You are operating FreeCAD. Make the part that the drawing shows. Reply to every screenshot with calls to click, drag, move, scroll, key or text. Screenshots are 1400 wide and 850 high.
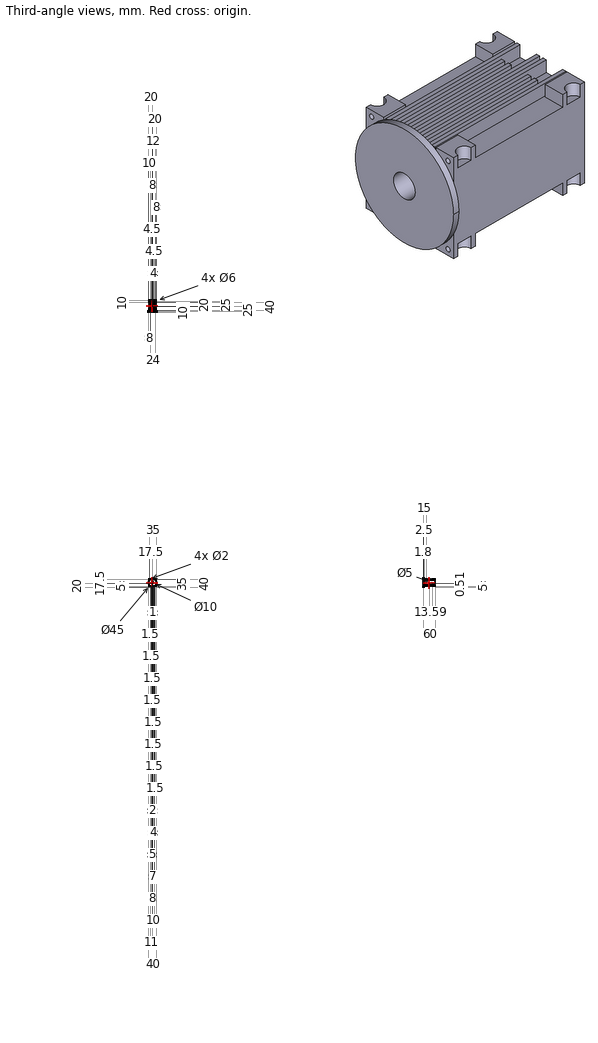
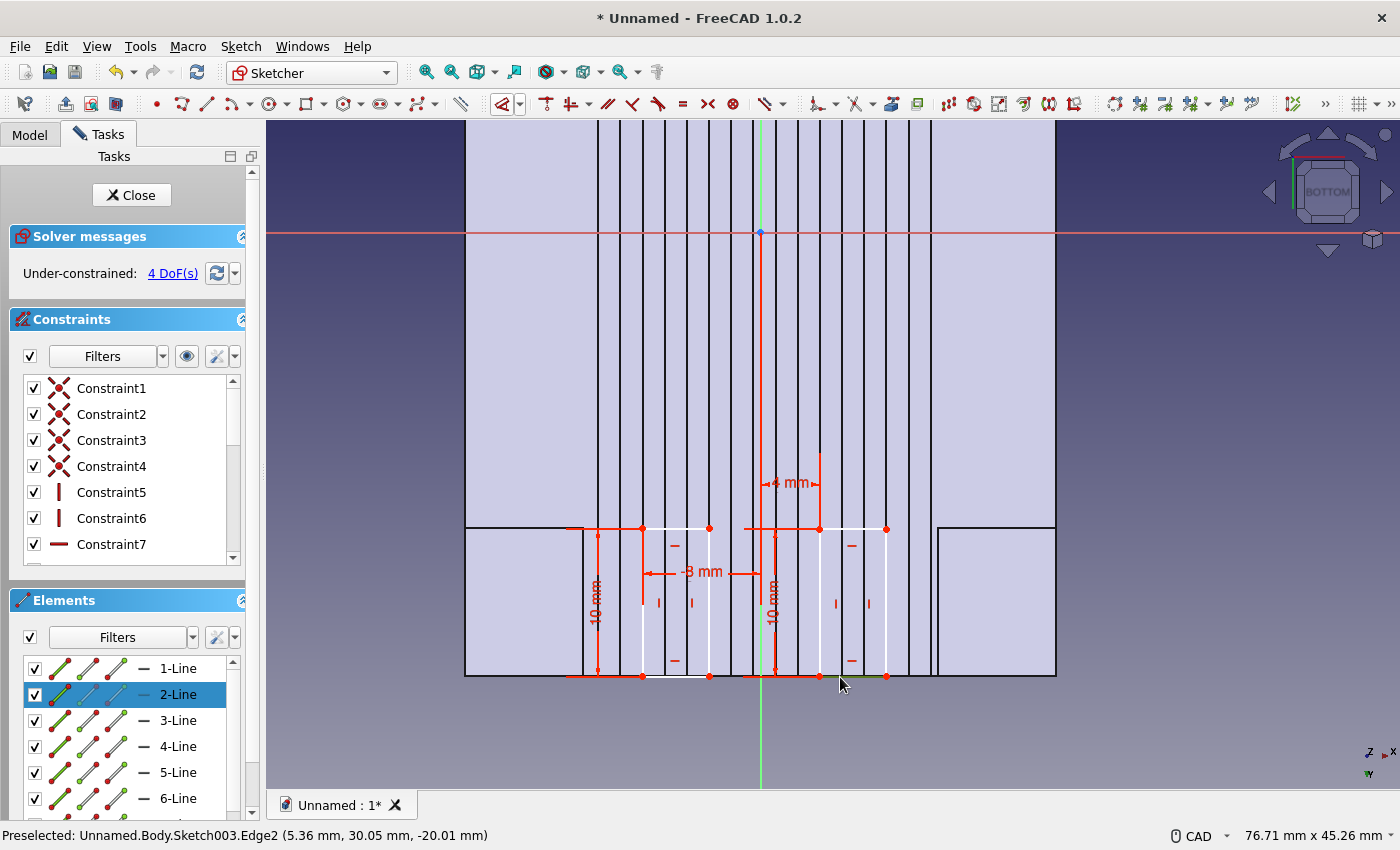
key(l)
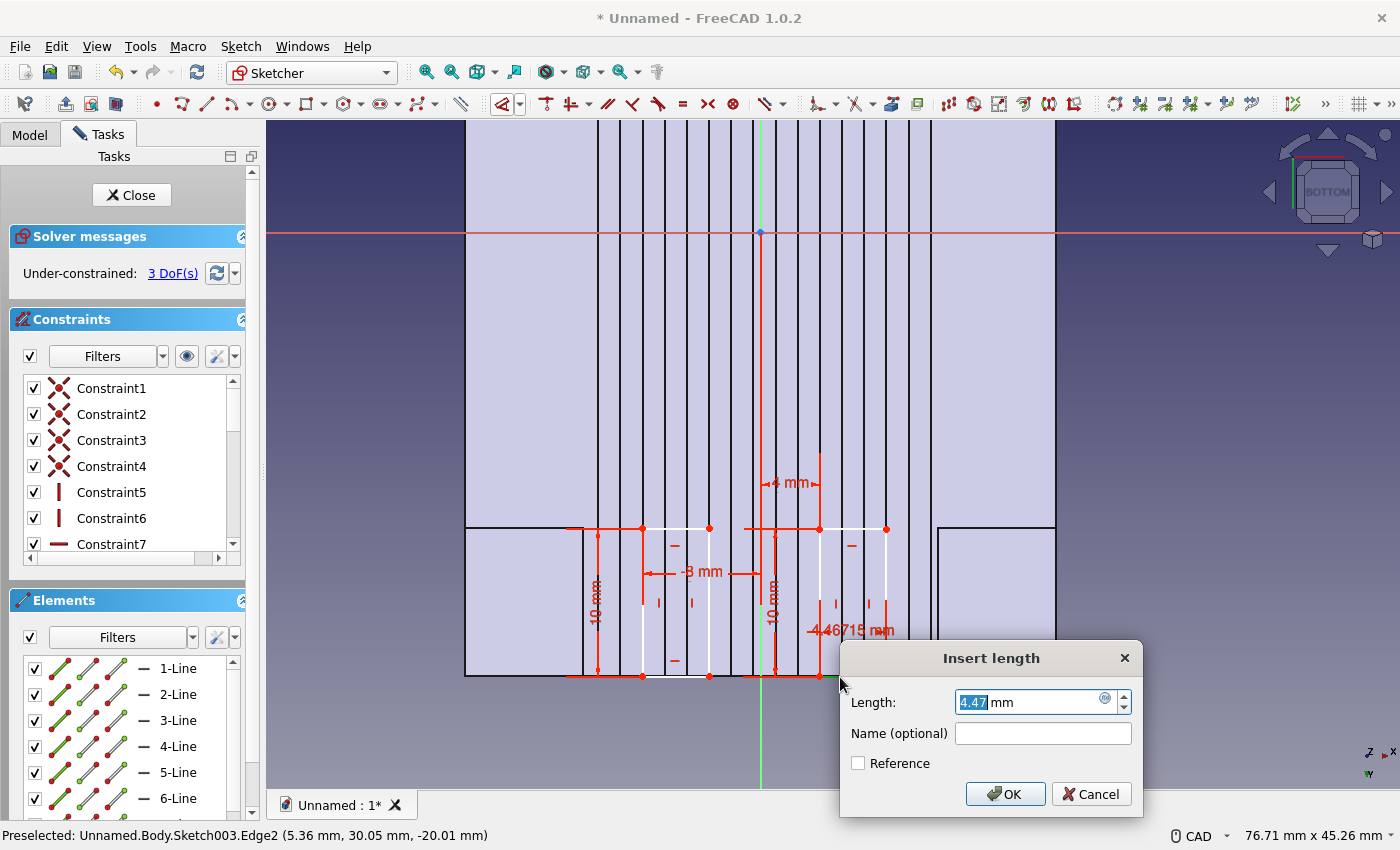
text(4.5)
key(Return)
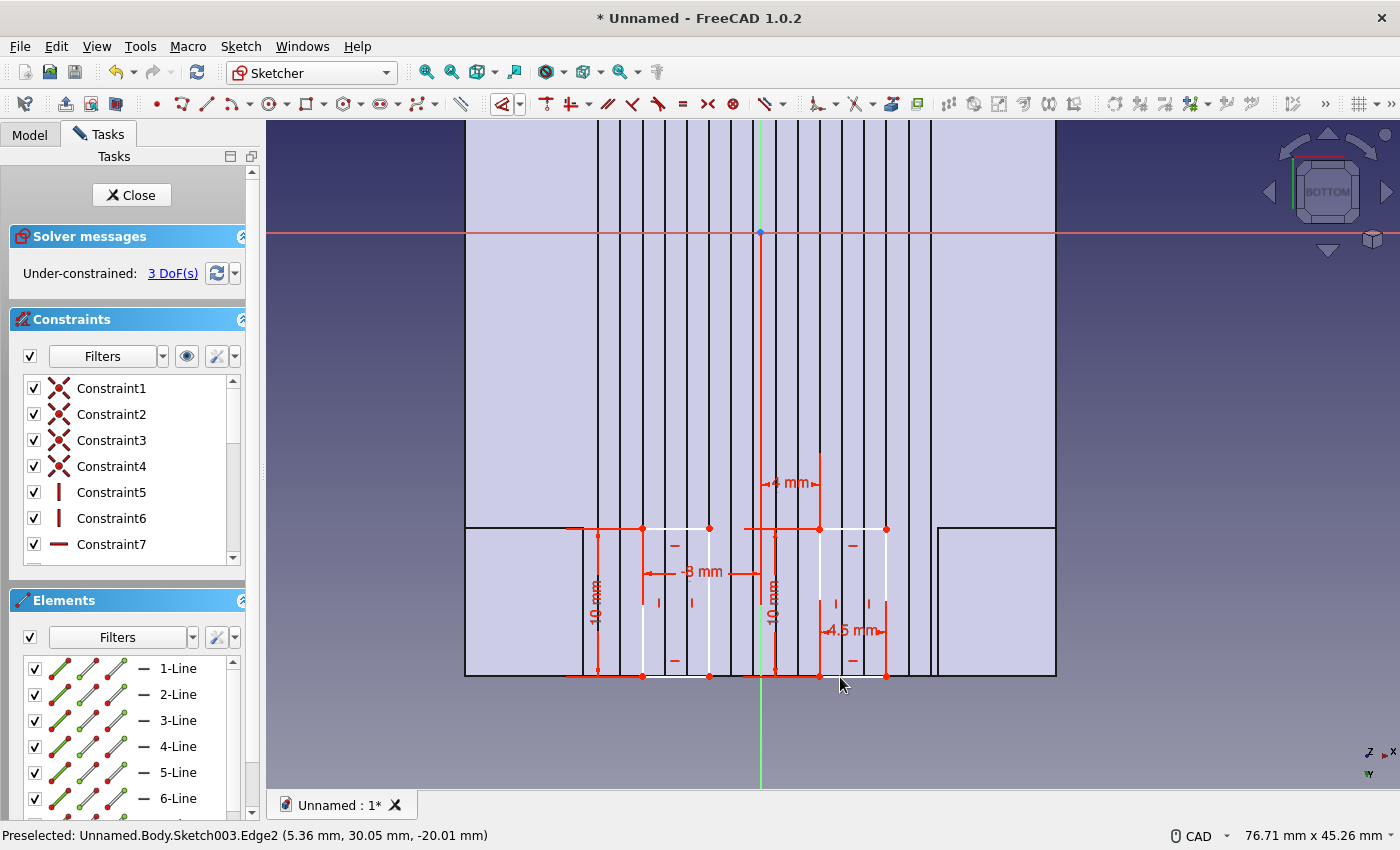
click(663, 677)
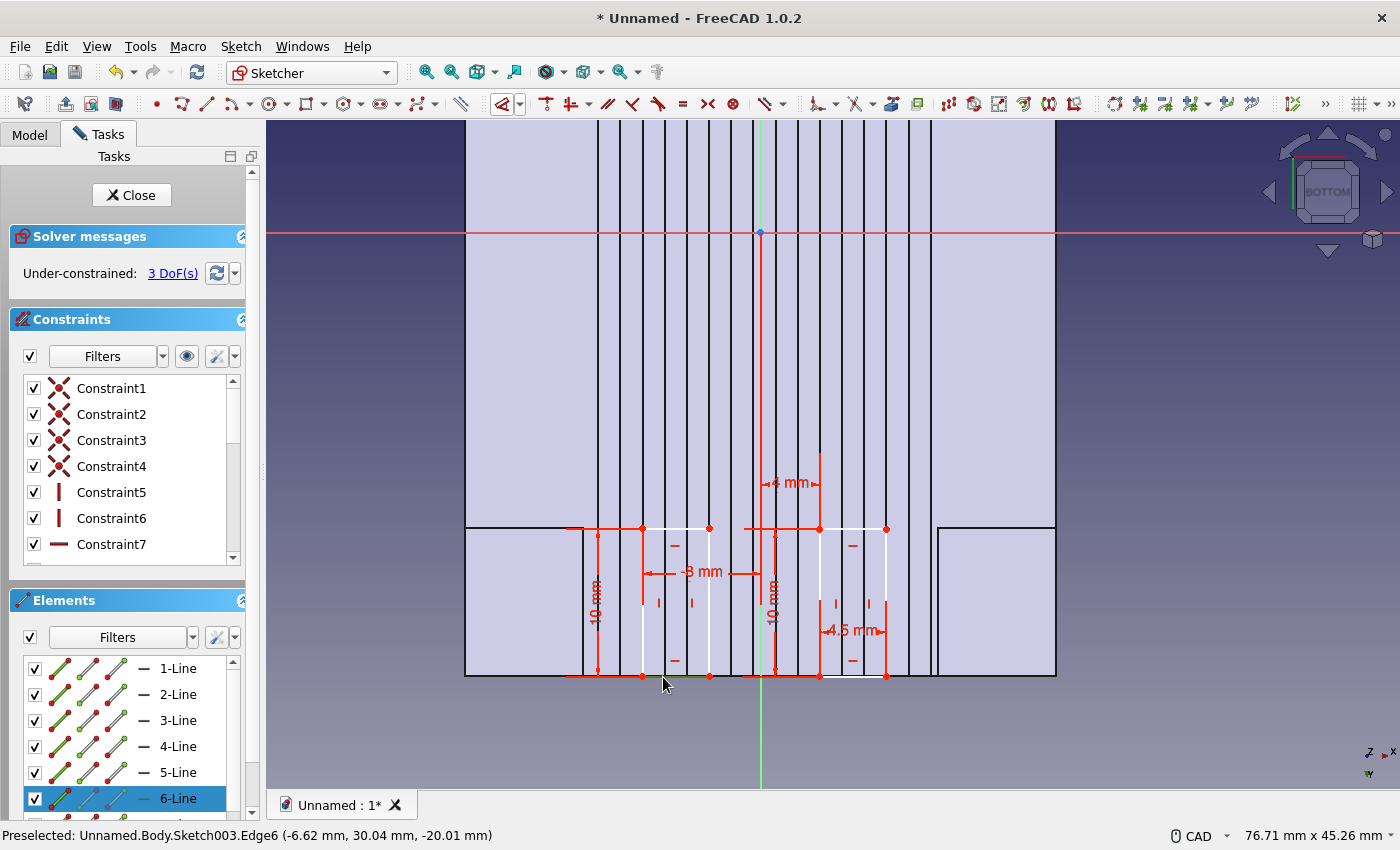
key(l)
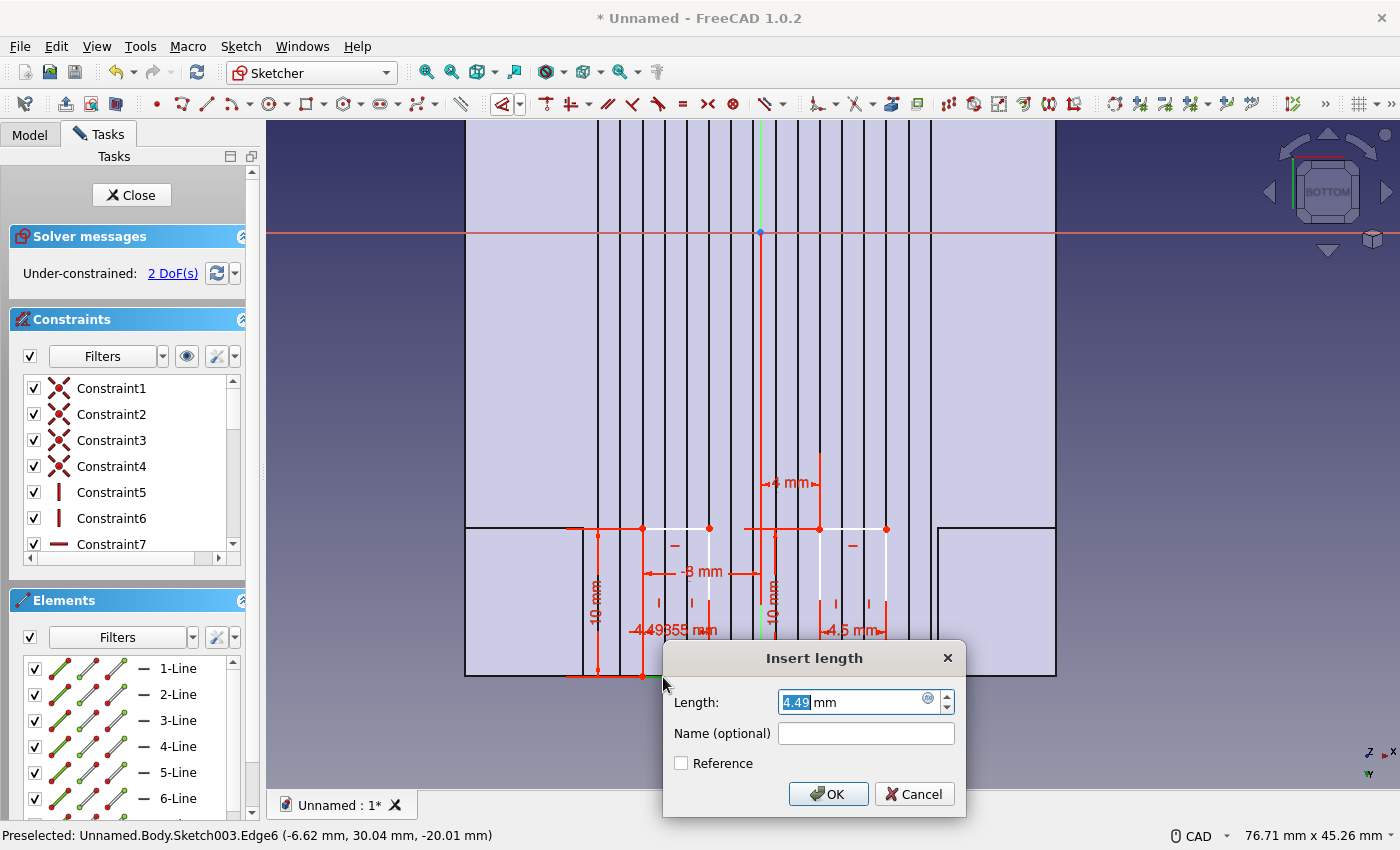
text(4.5)
key(Return)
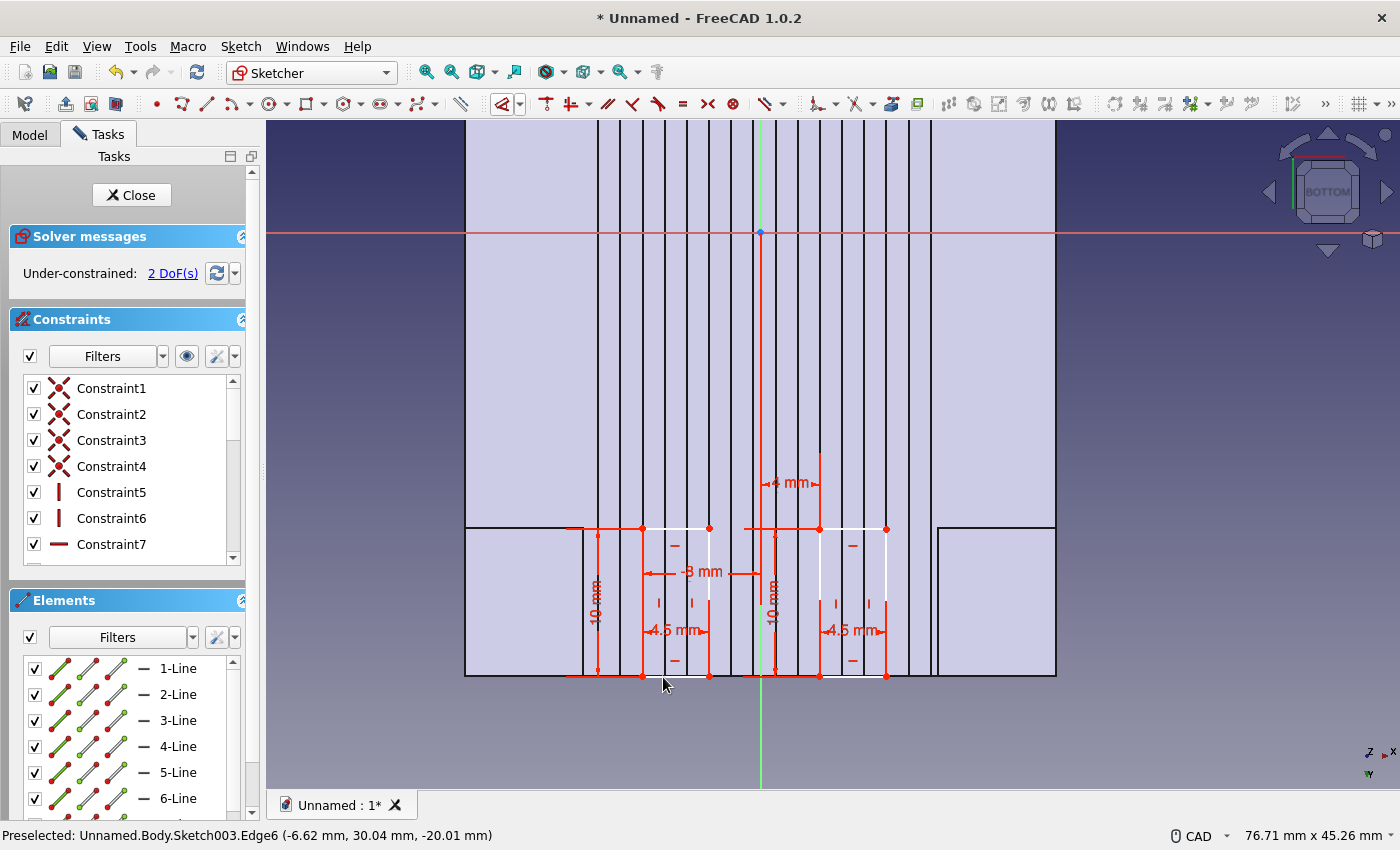
click(820, 529)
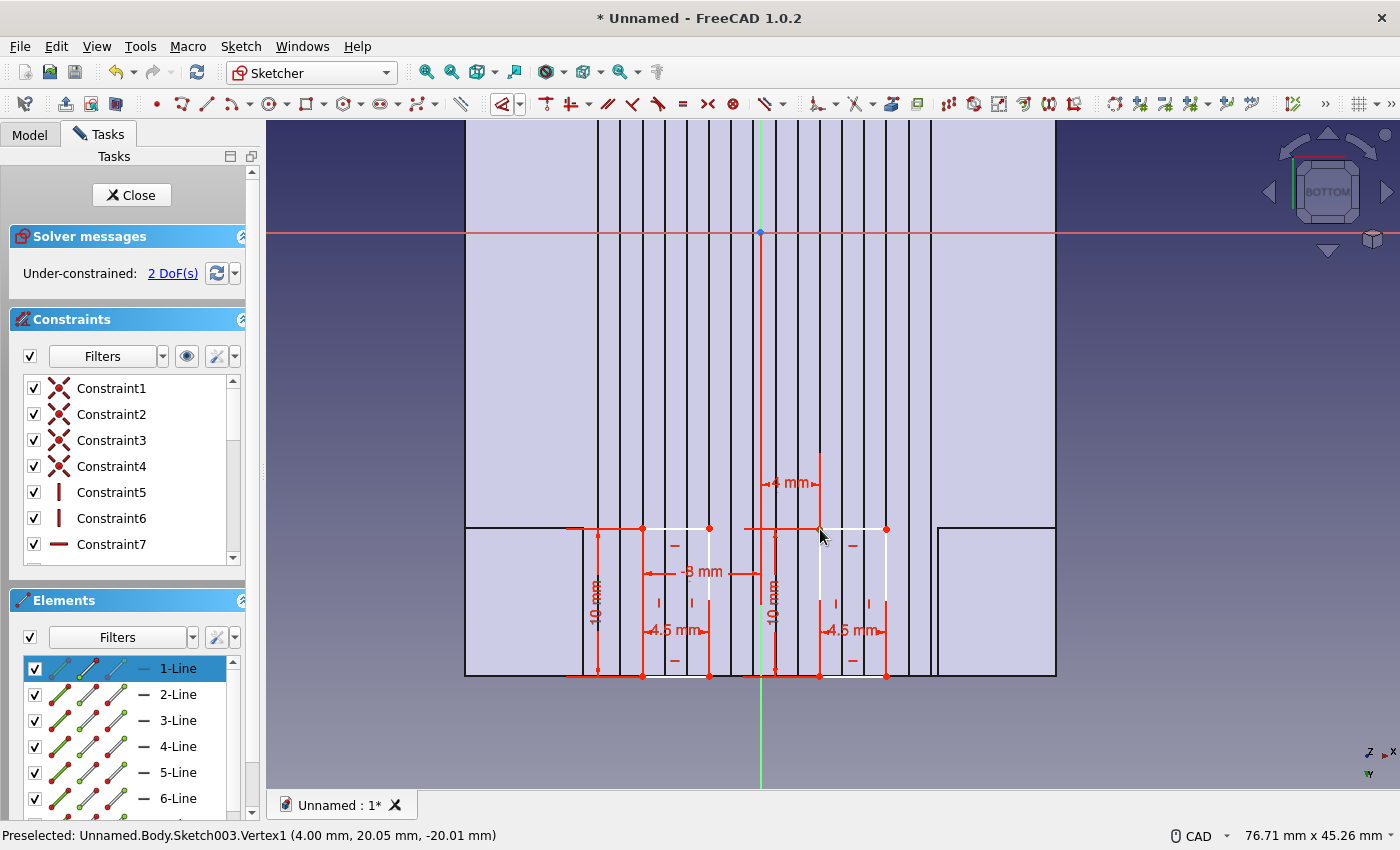
key(i)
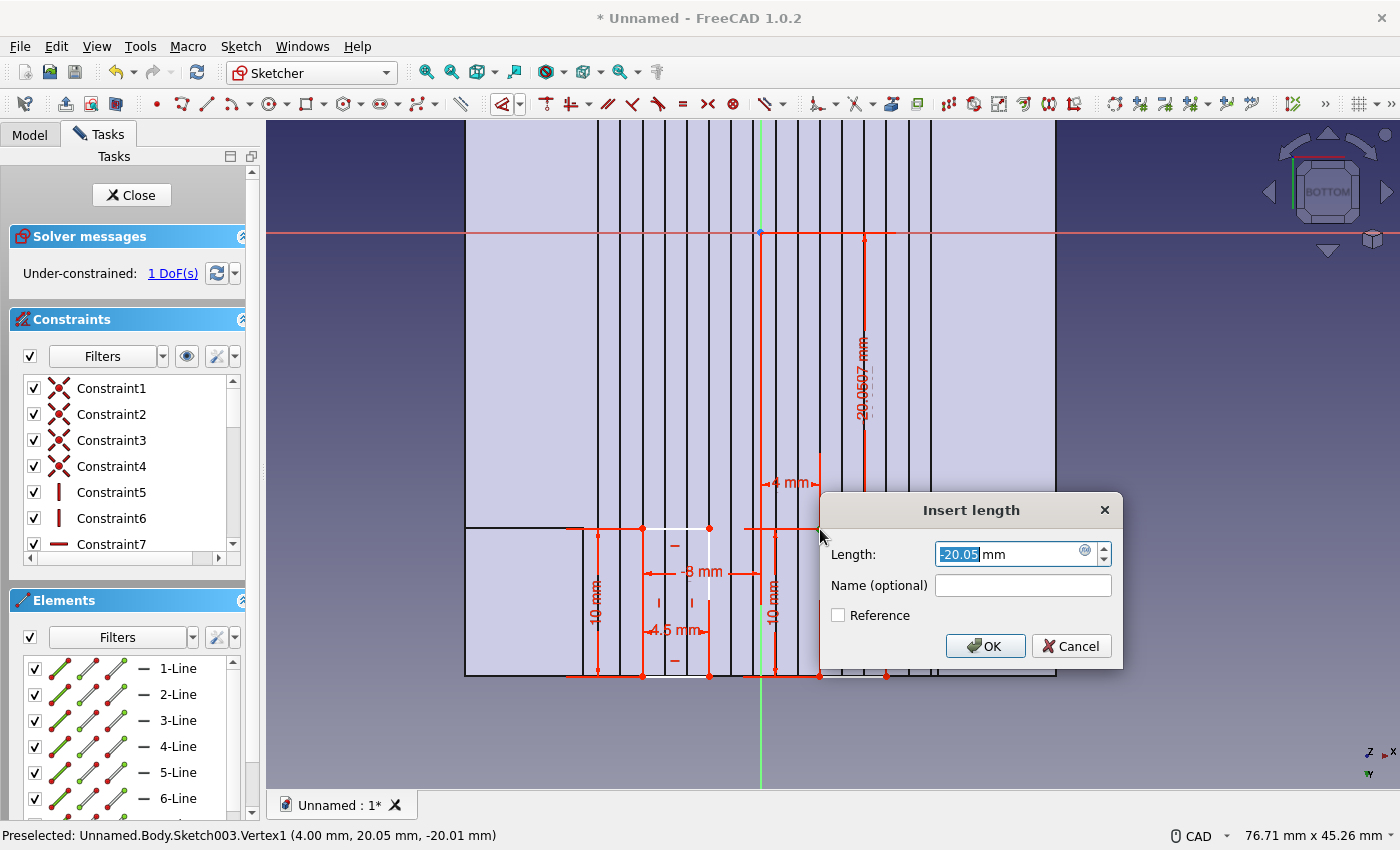
text(-20)
key(Return)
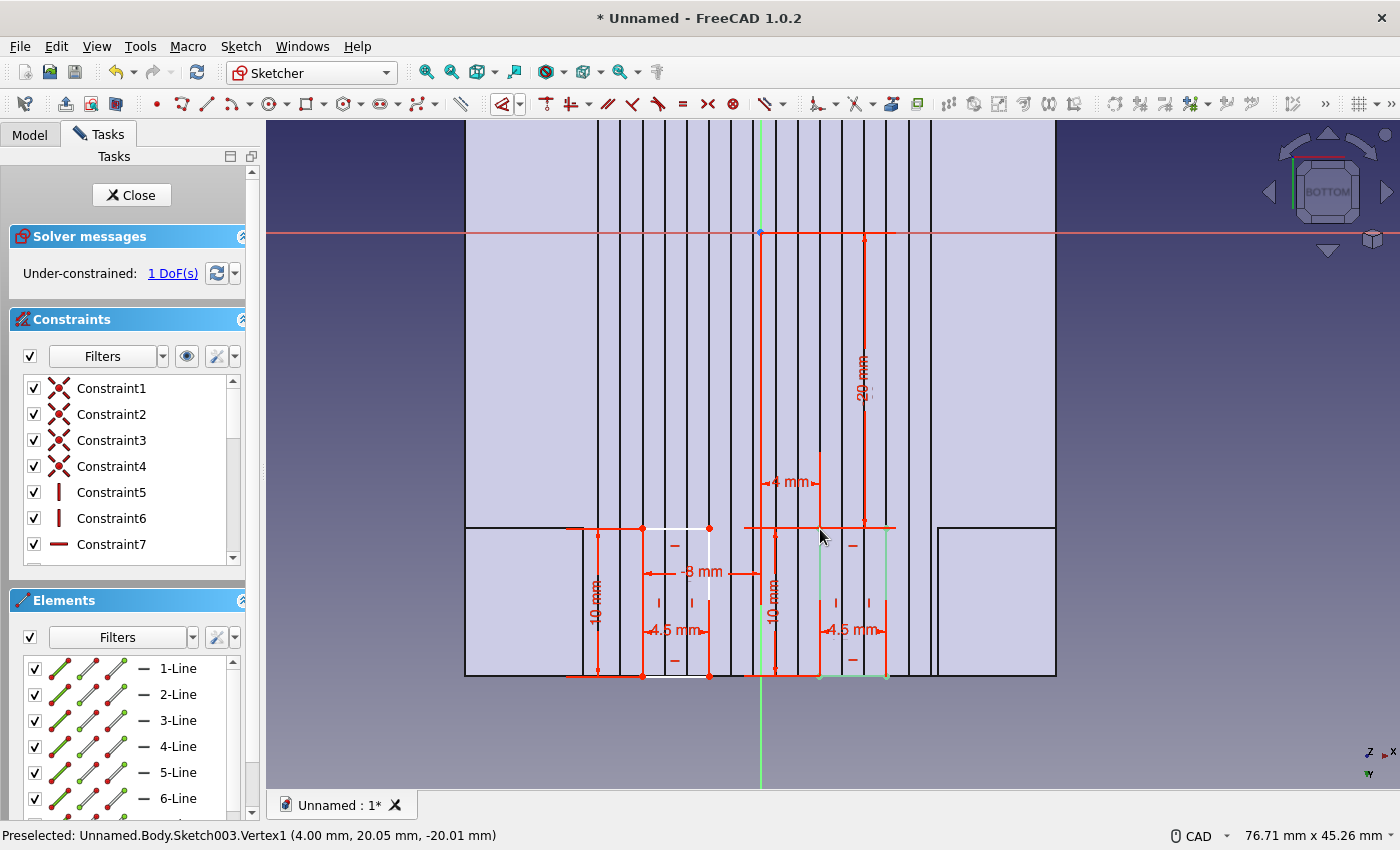
click(643, 529)